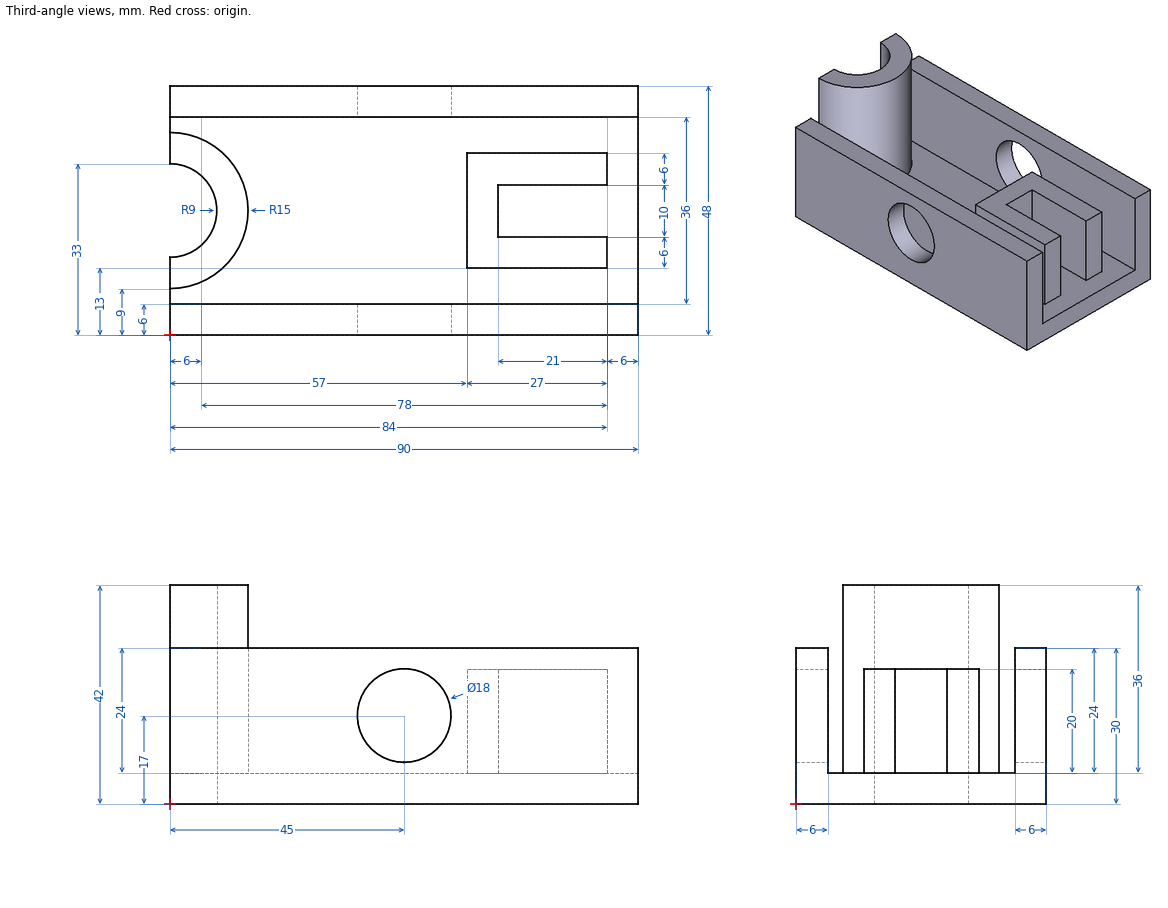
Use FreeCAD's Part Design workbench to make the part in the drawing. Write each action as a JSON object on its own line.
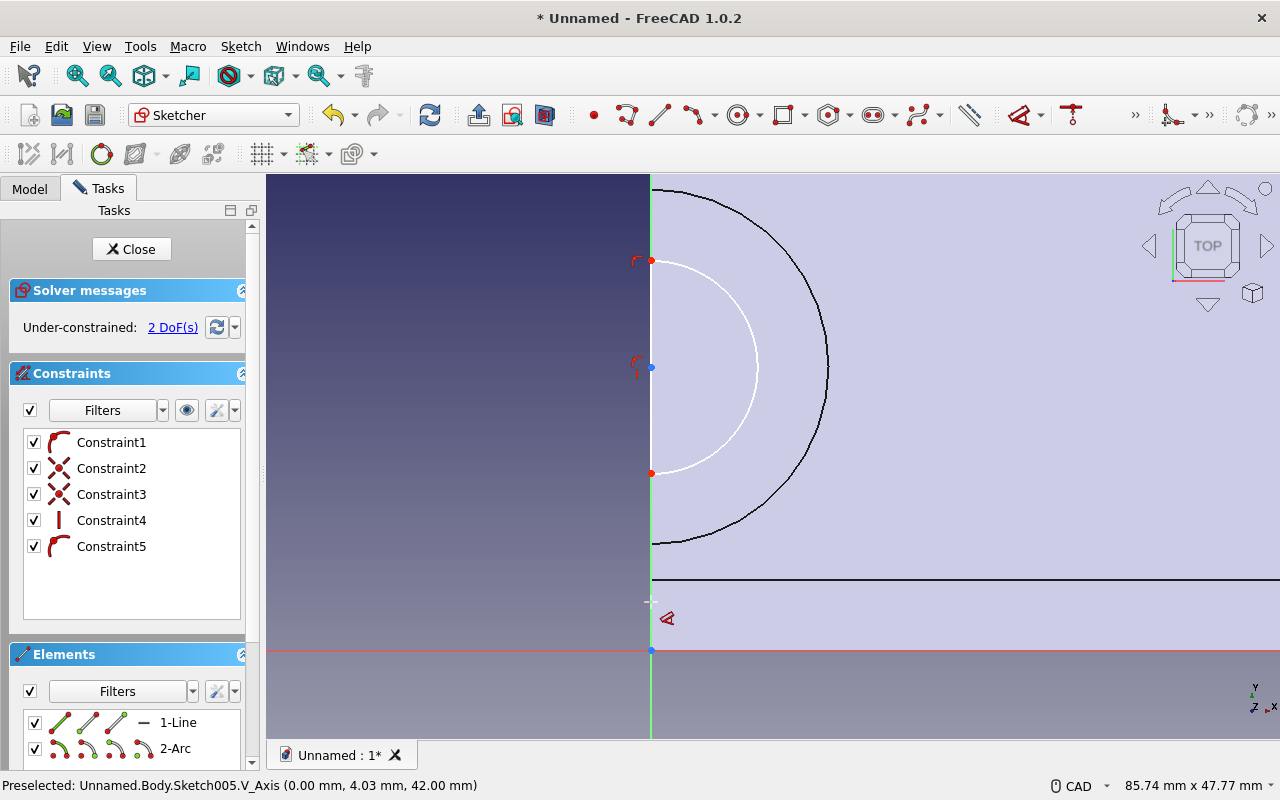
{"action": "left_click", "coordinate": [737, 430]}
{"action": "left_click", "coordinate": [763, 449]}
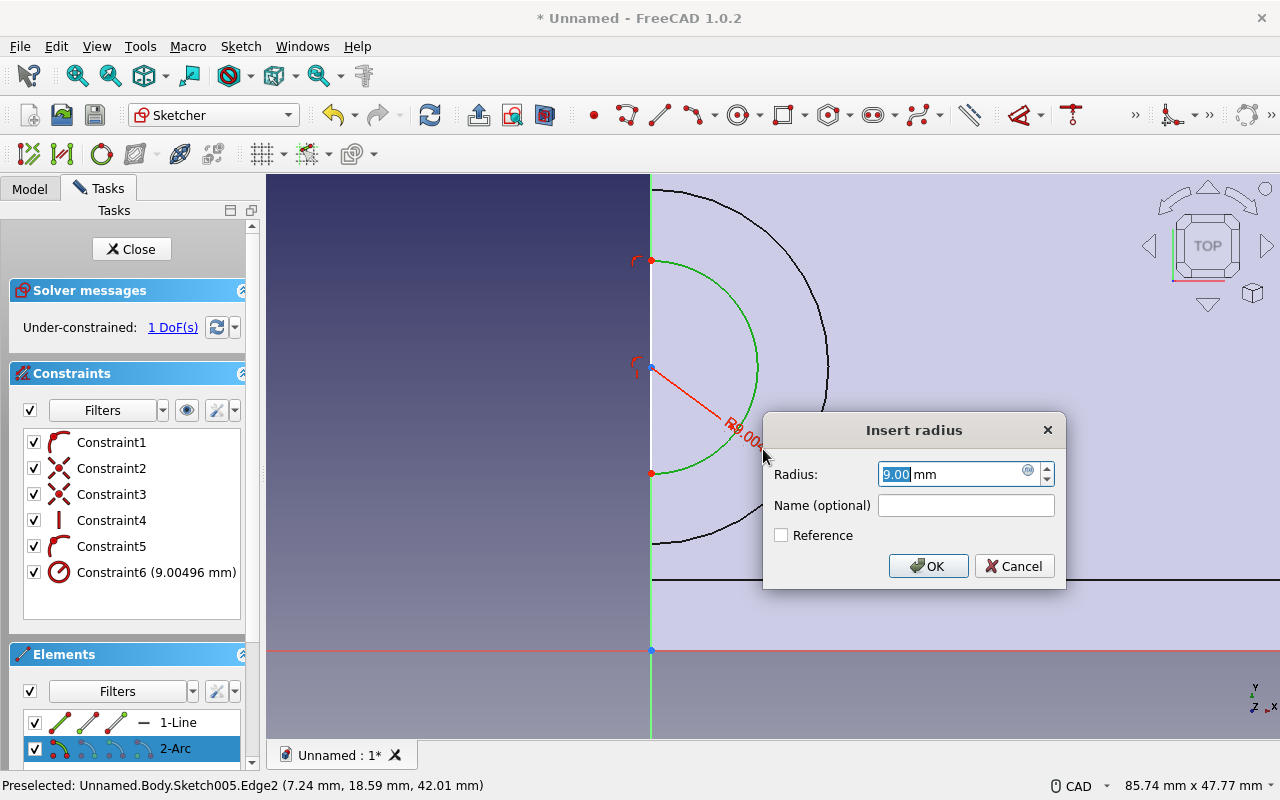
{"action": "type", "text": "9"}
{"action": "key", "text": "Return"}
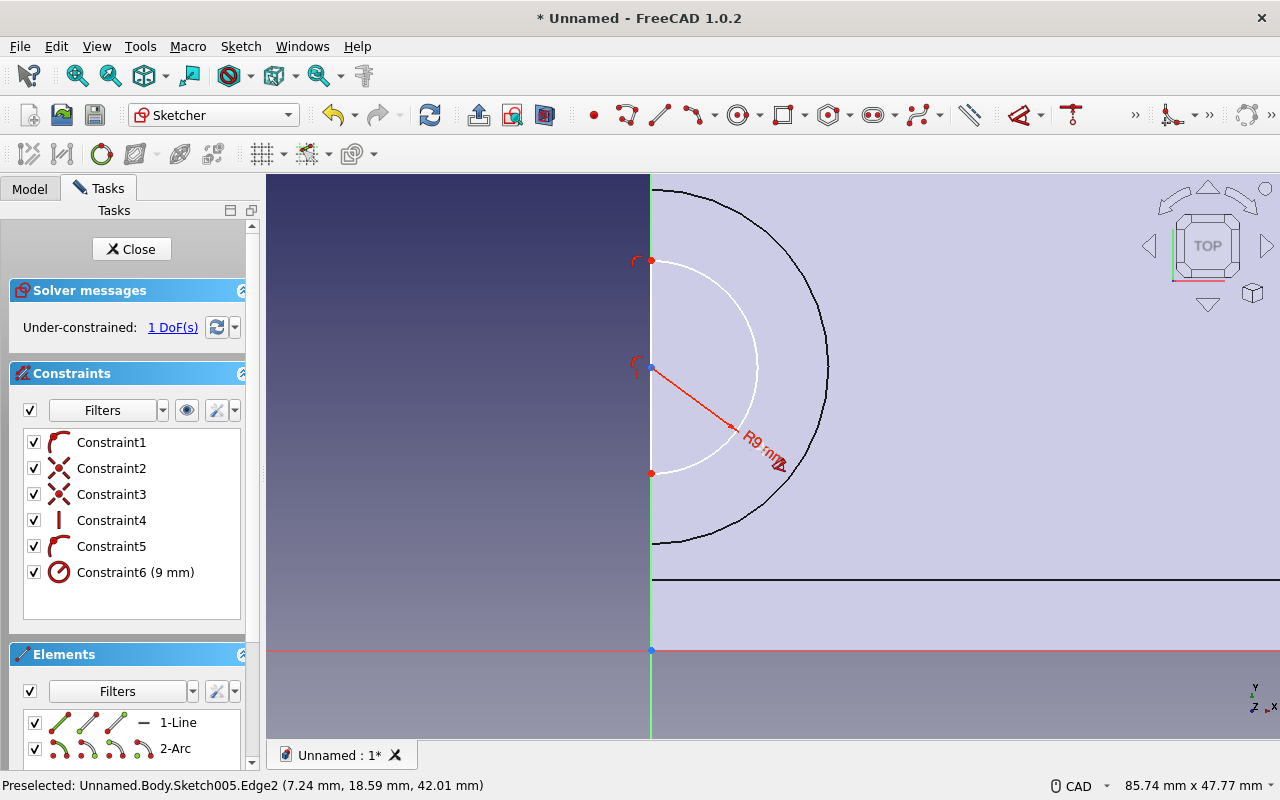
{"action": "left_click", "coordinate": [651, 261]}
{"action": "left_click", "coordinate": [617, 456]}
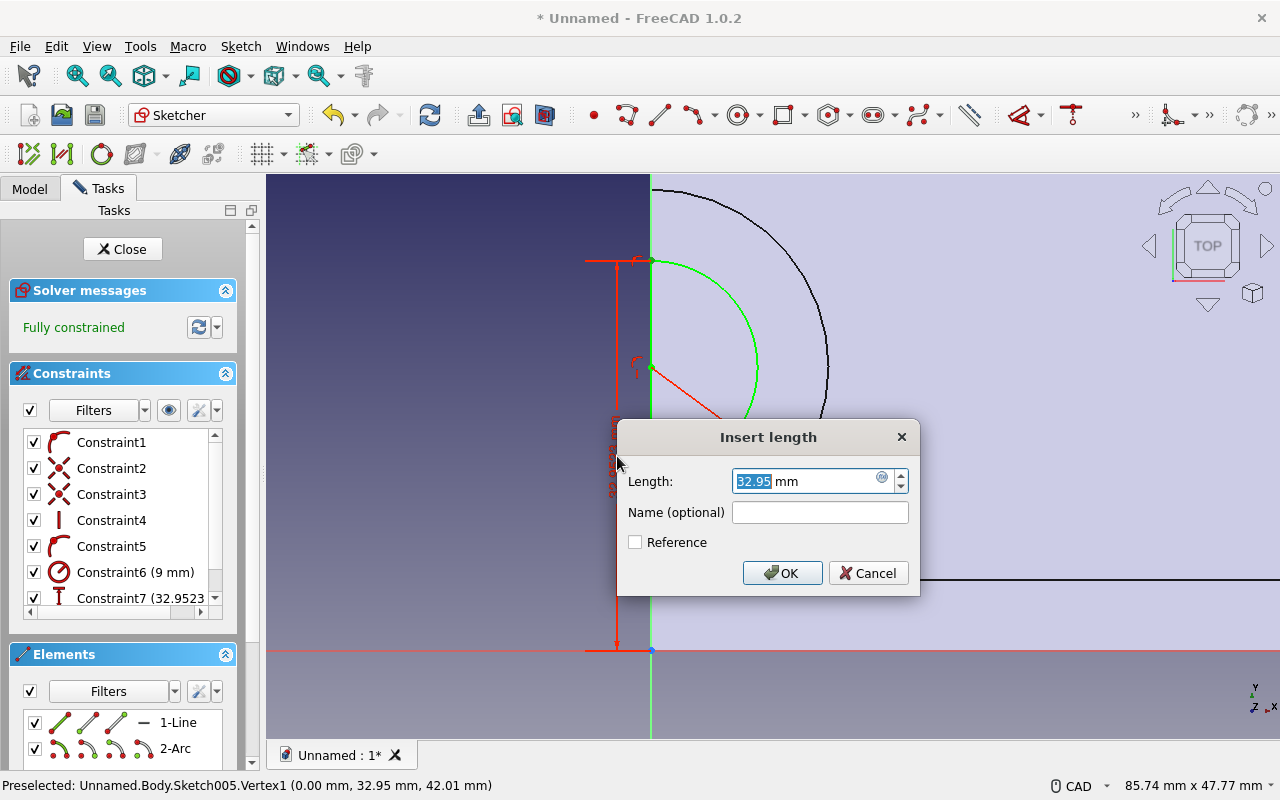
{"action": "type", "text": "33"}
{"action": "key", "text": "Return"}
{"action": "key", "text": "Escape"}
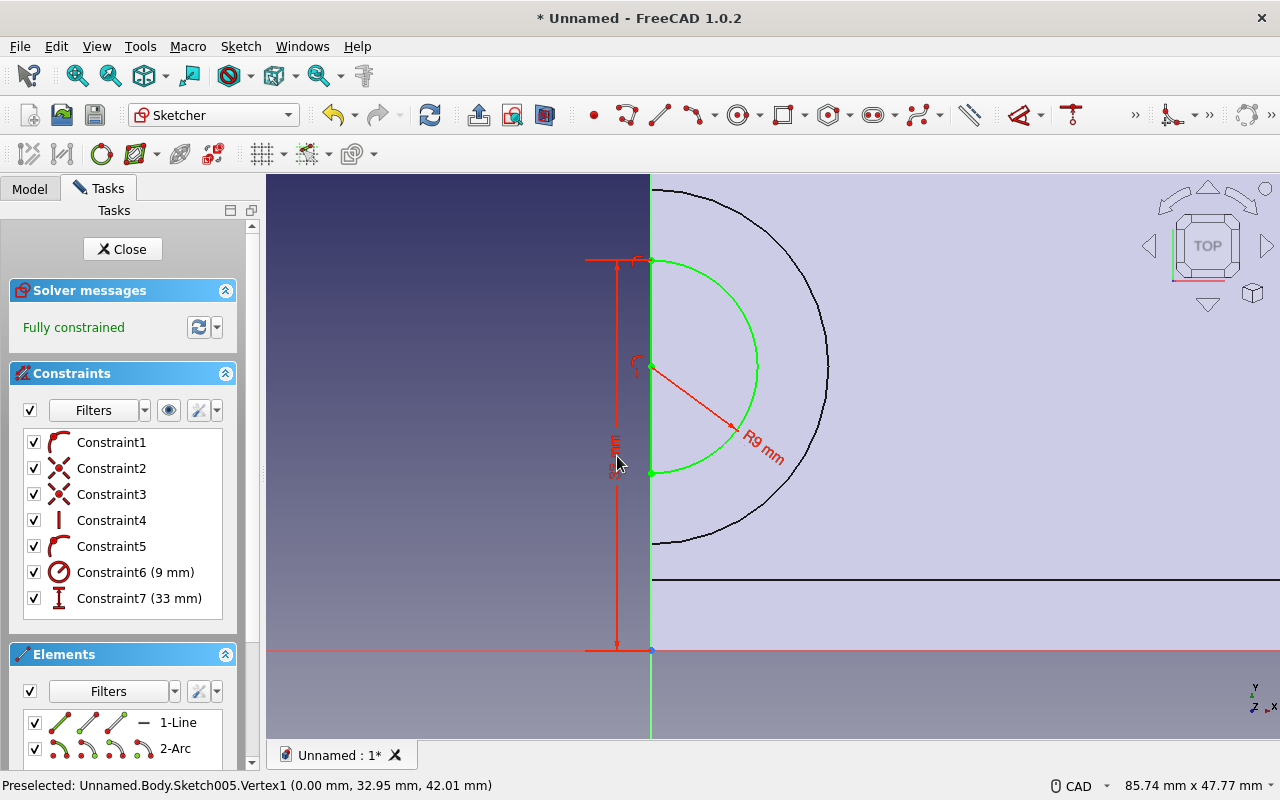
{"action": "left_click", "coordinate": [123, 249]}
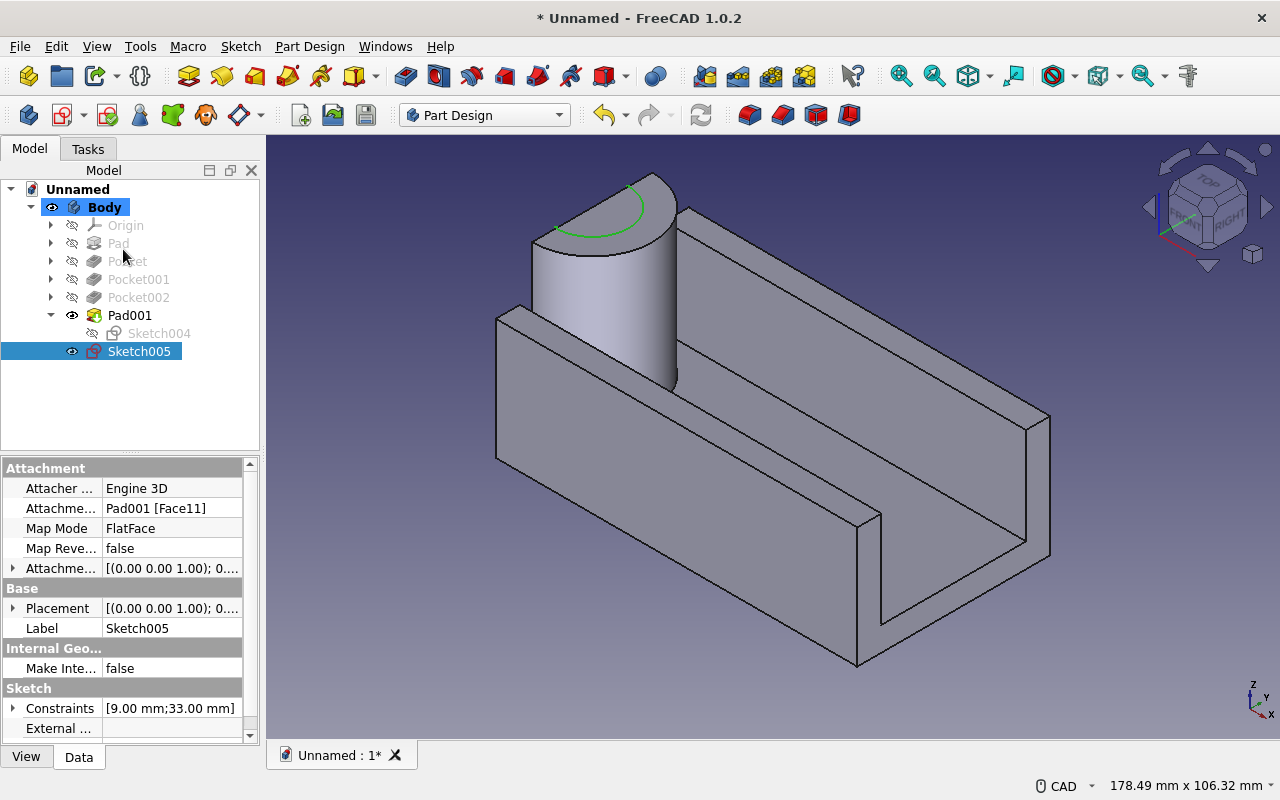
{"action": "left_click", "coordinate": [406, 76]}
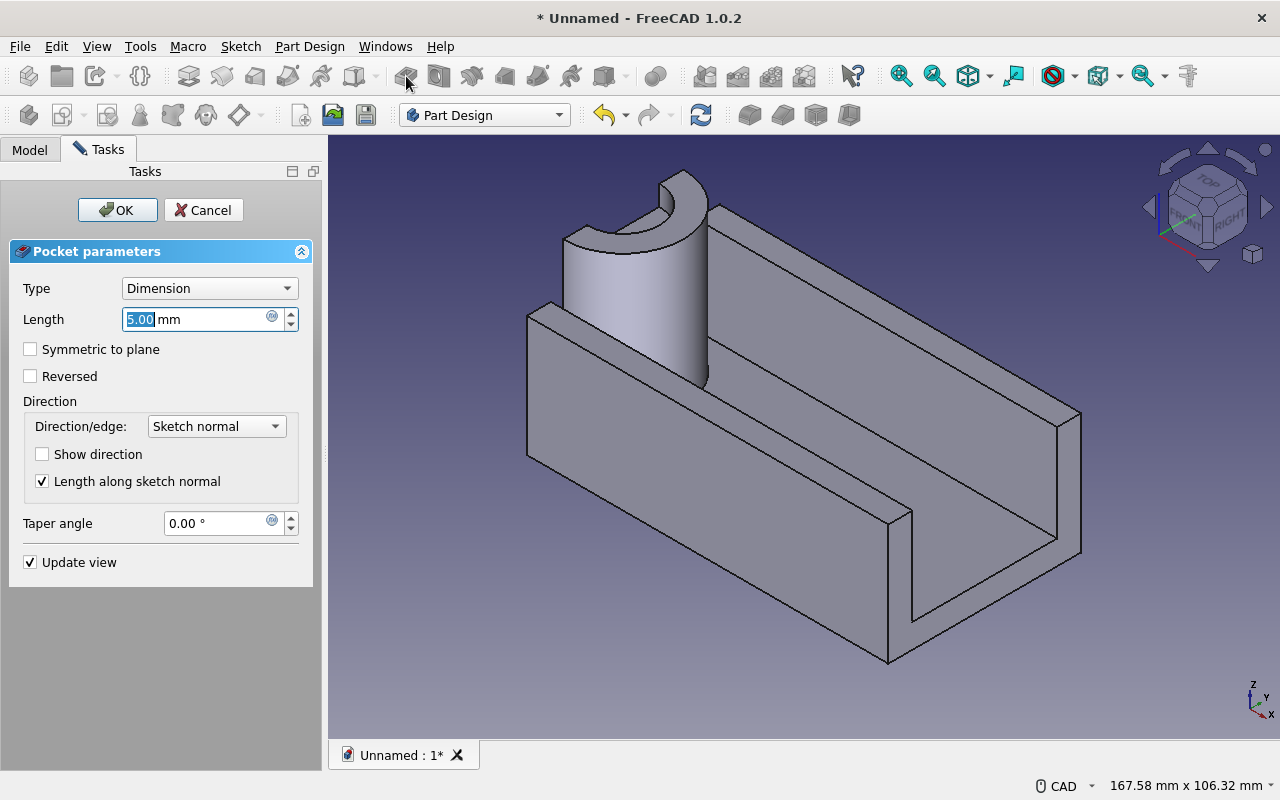
{"action": "type", "text": "42"}
{"action": "key", "text": "Tab"}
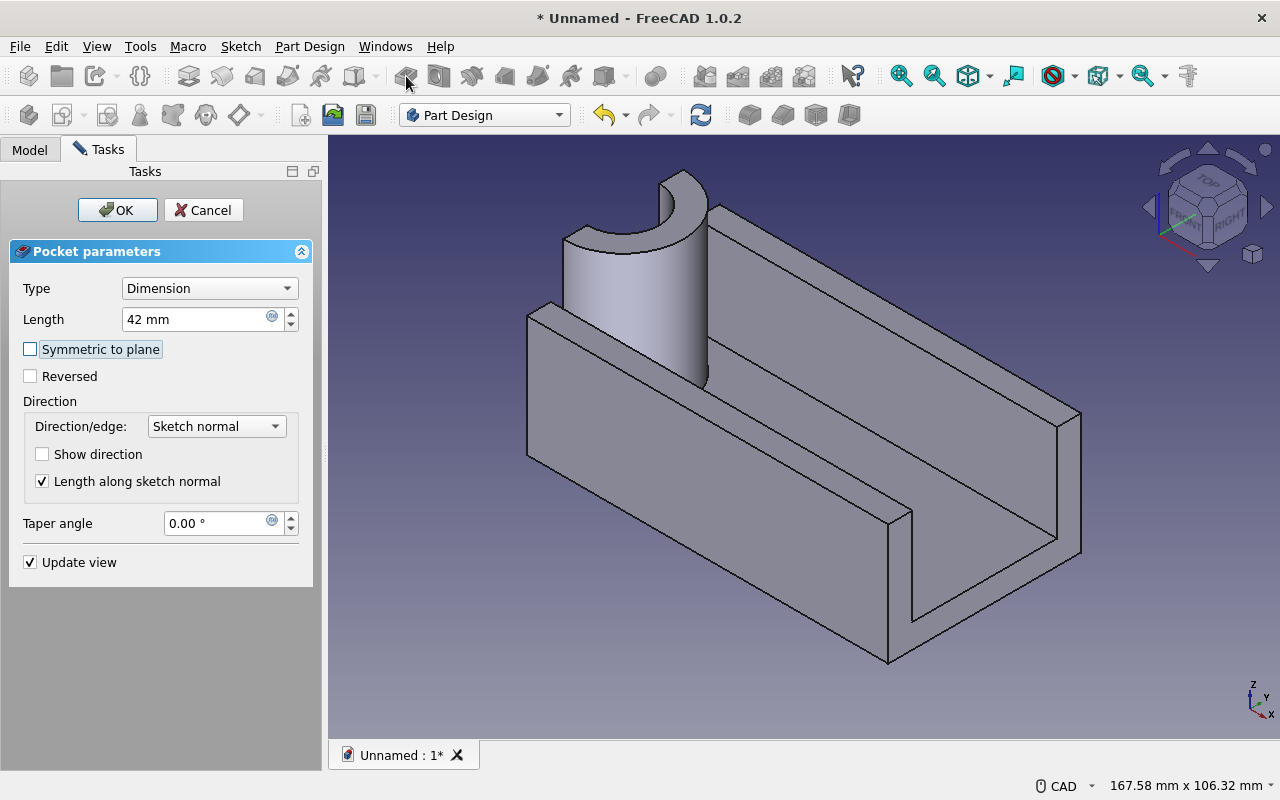
{"action": "left_click", "coordinate": [118, 210]}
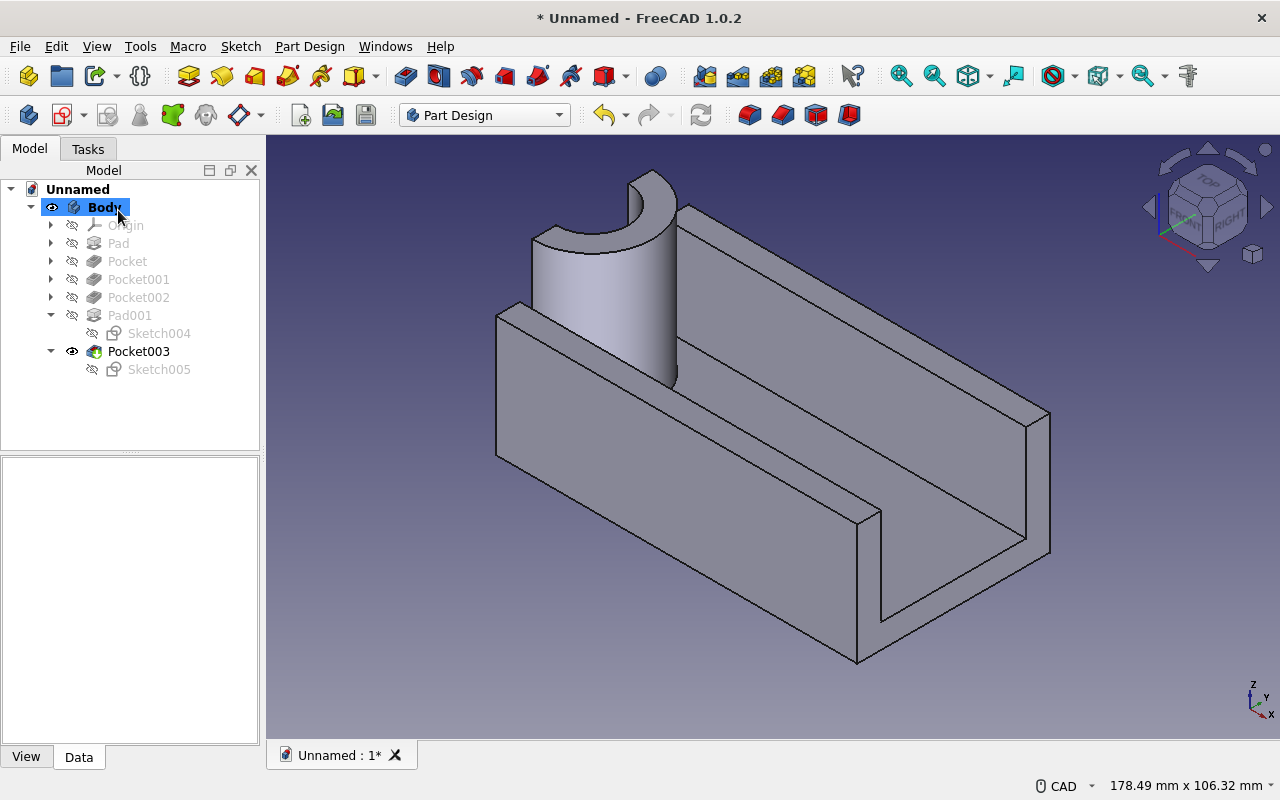
{"action": "left_click", "coordinate": [62, 116]}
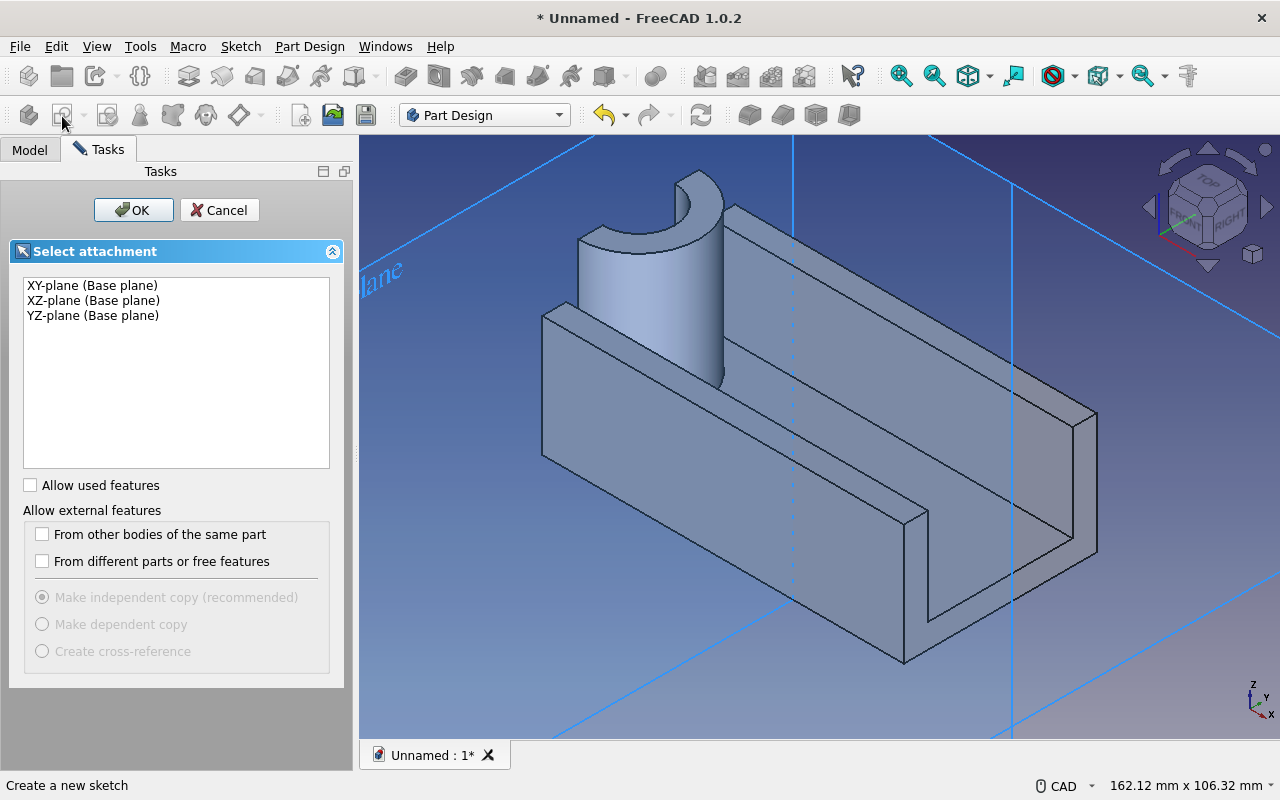
{"action": "left_click", "coordinate": [84, 300]}